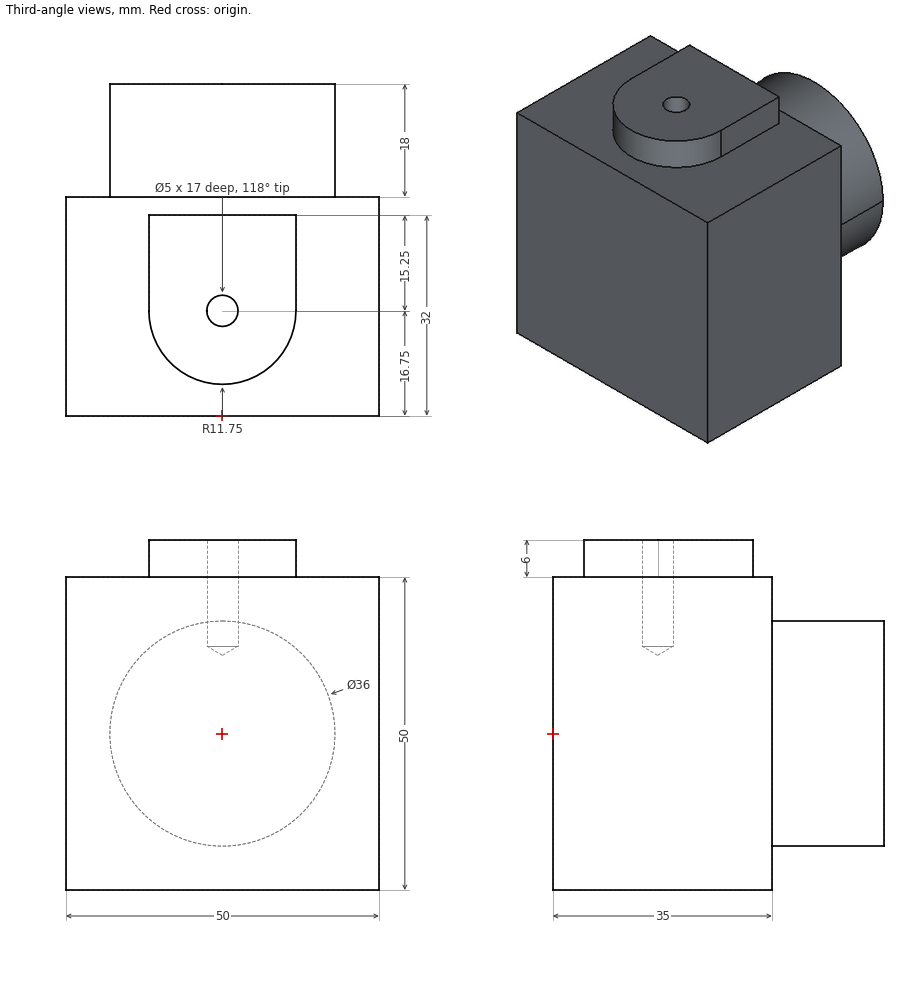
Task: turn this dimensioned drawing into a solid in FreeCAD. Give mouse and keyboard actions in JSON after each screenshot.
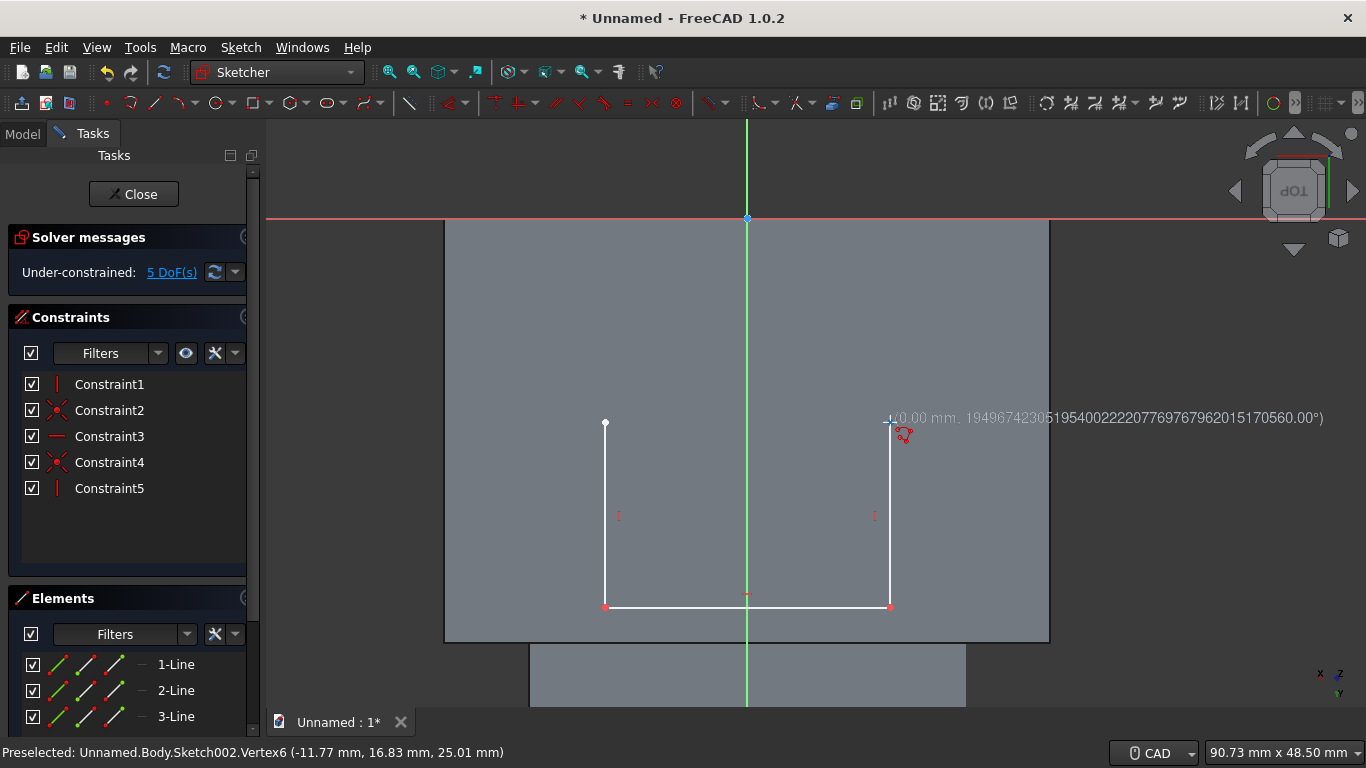
{"action": "key", "text": "g 3 a"}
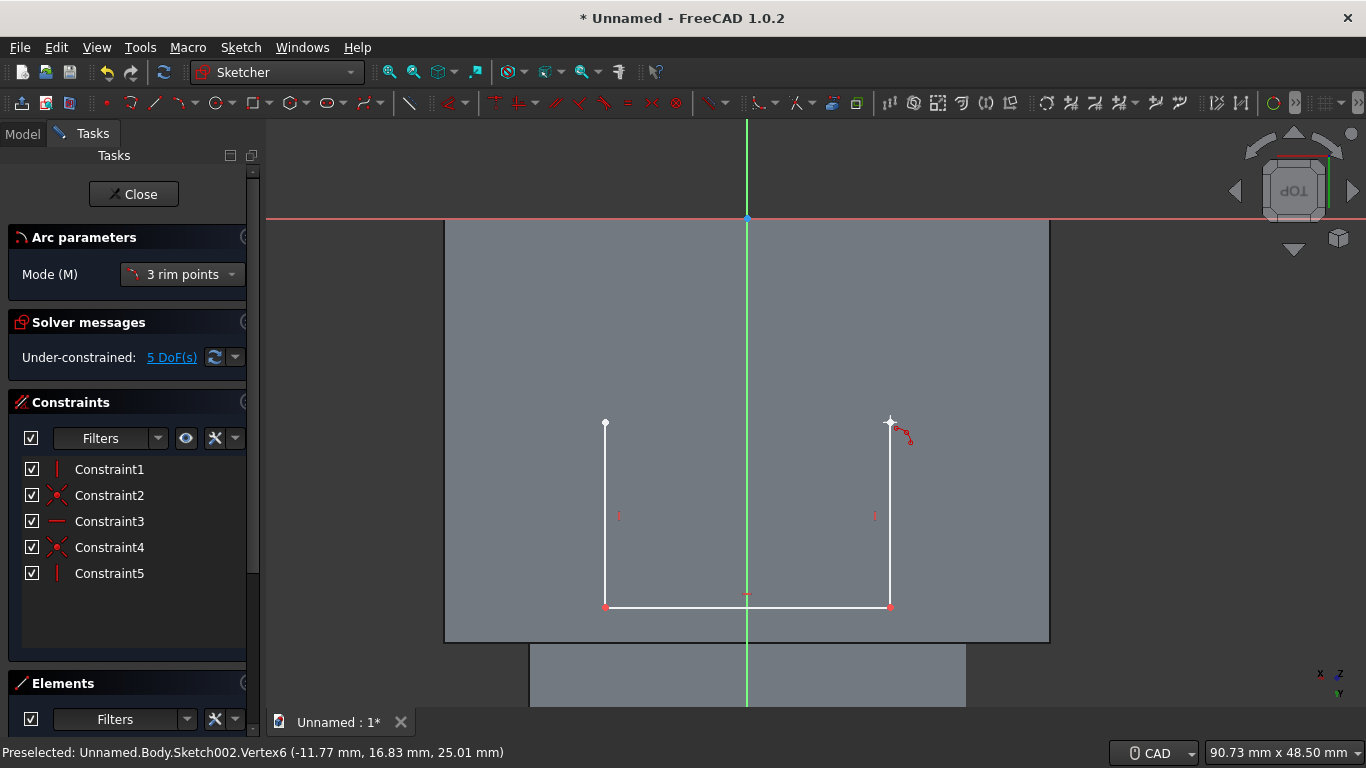
{"action": "left_click", "coordinate": [890, 423]}
{"action": "left_click", "coordinate": [605, 423]}
{"action": "left_click", "coordinate": [791, 287]}
{"action": "key", "text": "Escape"}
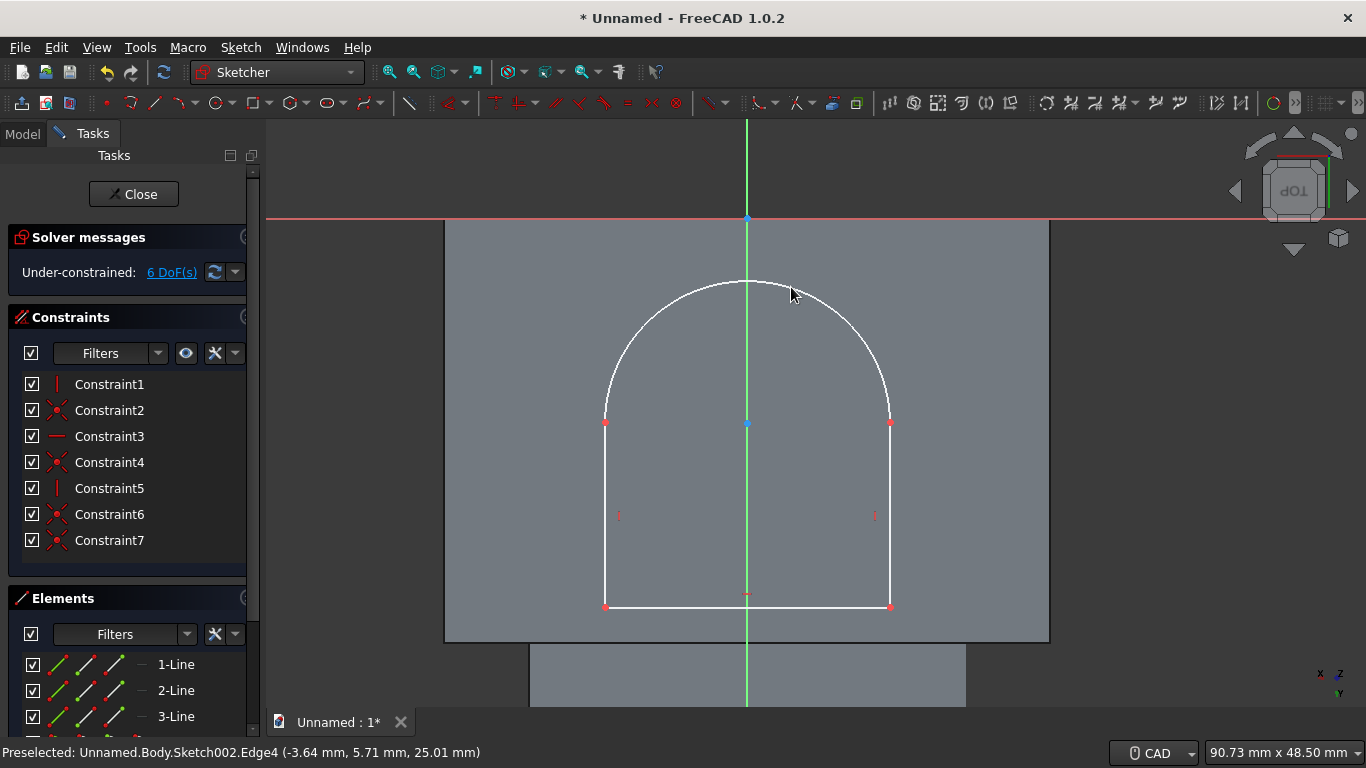
{"action": "left_click", "coordinate": [605, 479]}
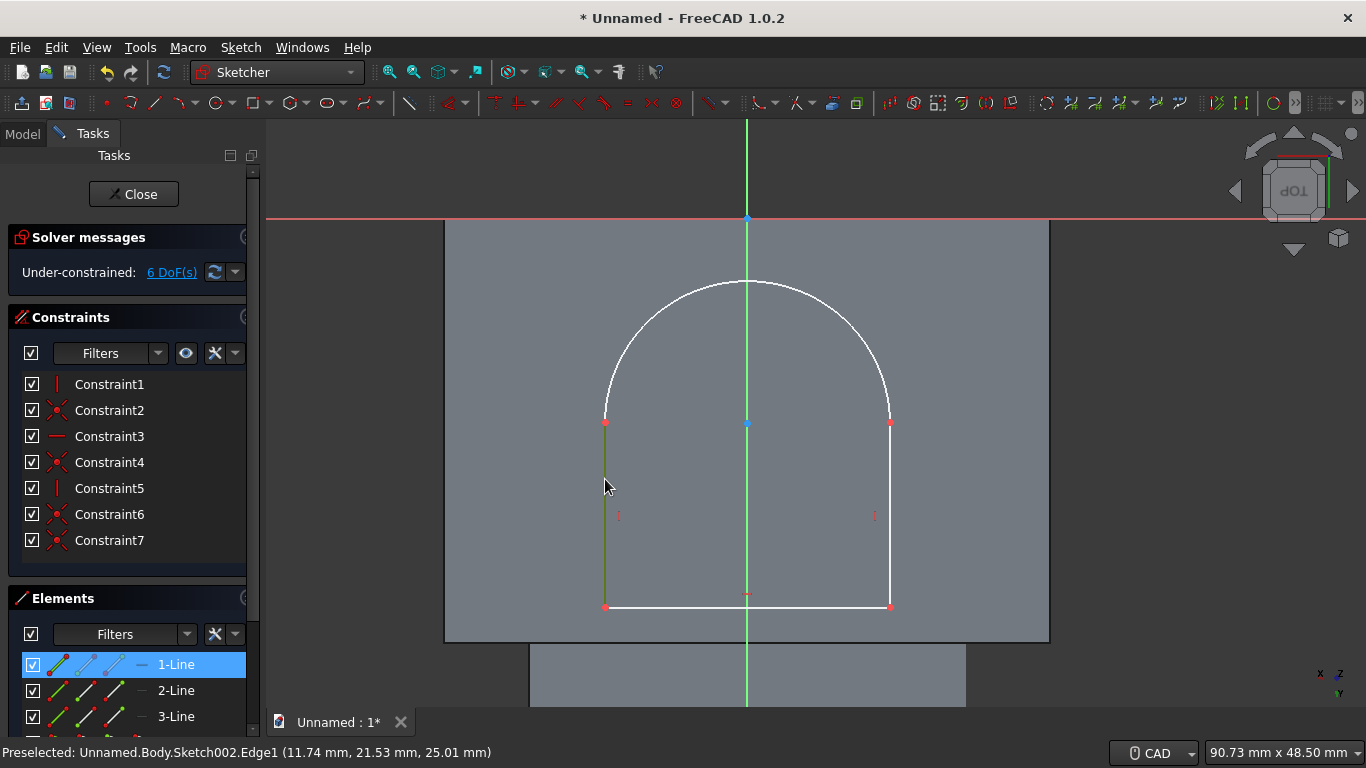
{"action": "left_click", "coordinate": [831, 308]}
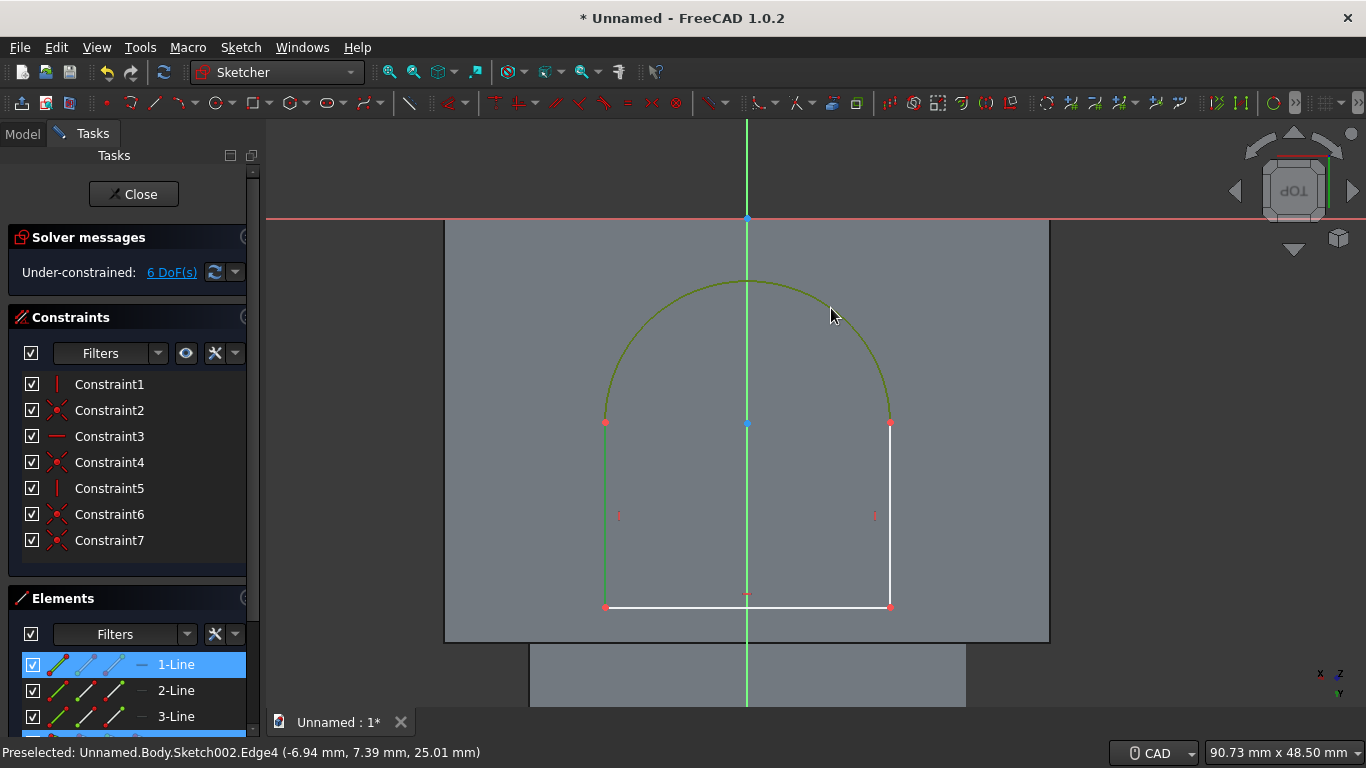
{"action": "key", "text": "t"}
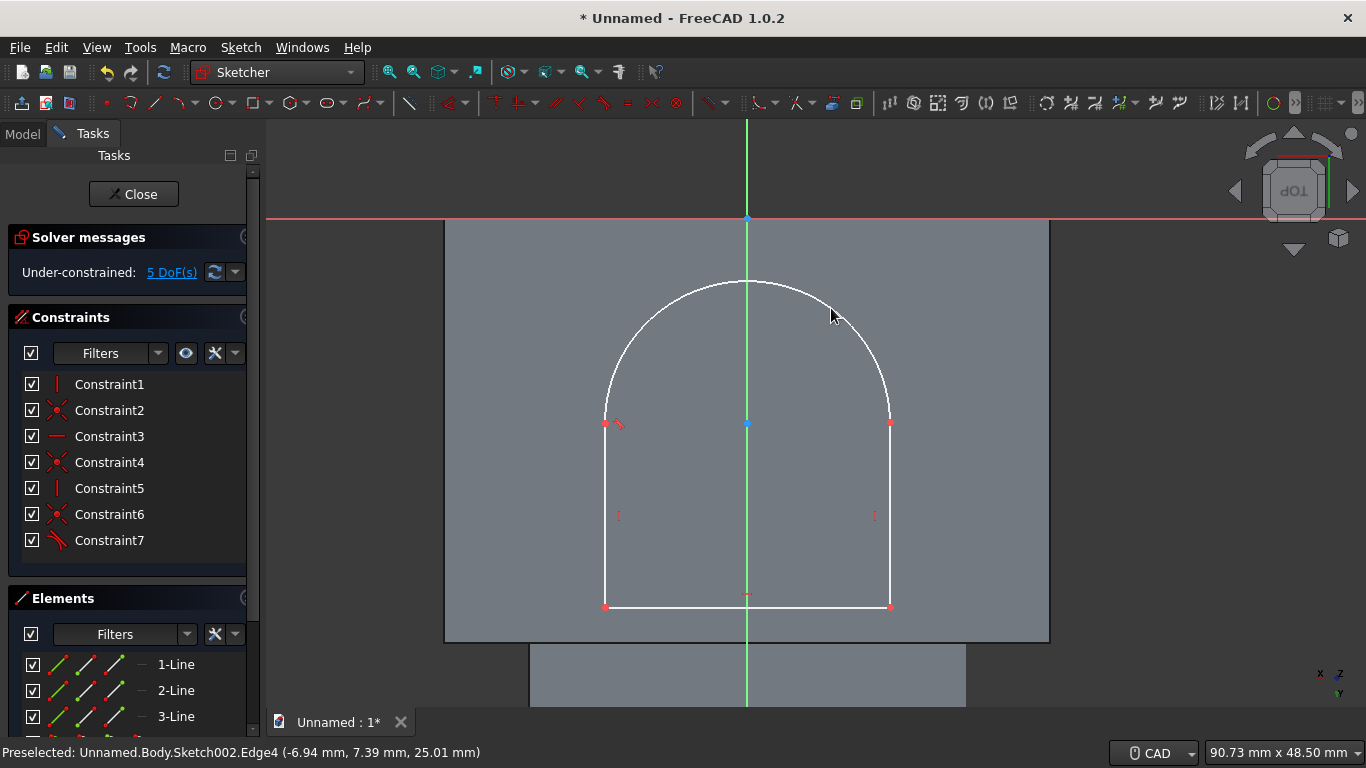
{"action": "left_click", "coordinate": [890, 553]}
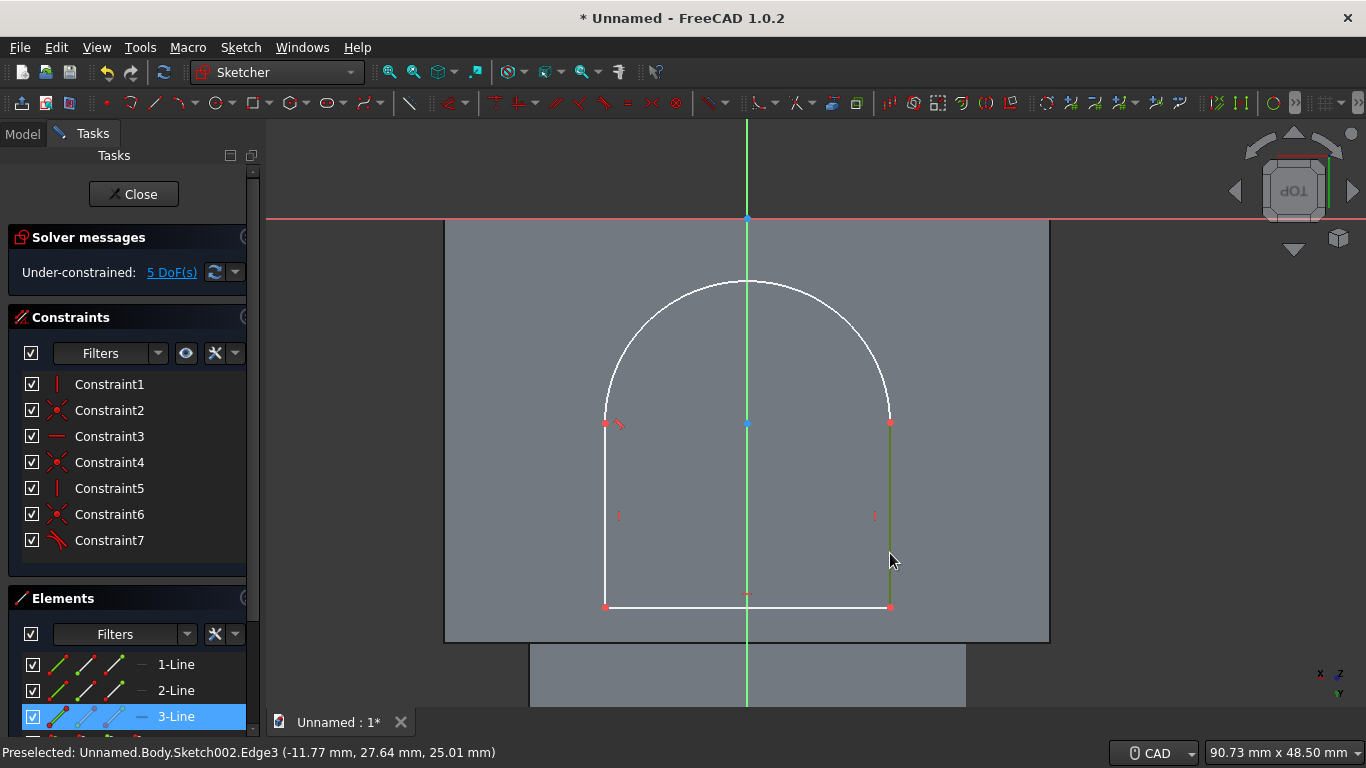
{"action": "left_click", "coordinate": [831, 308]}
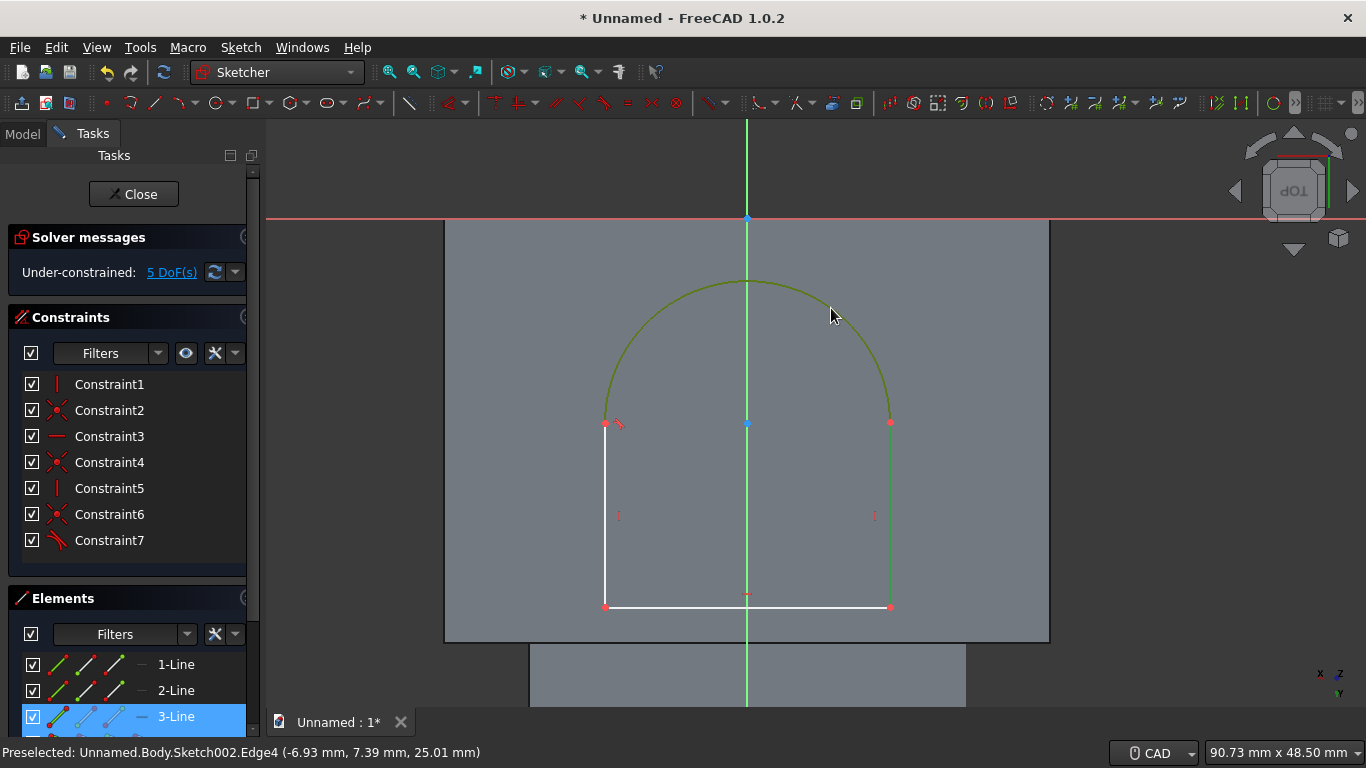
{"action": "key", "text": "t"}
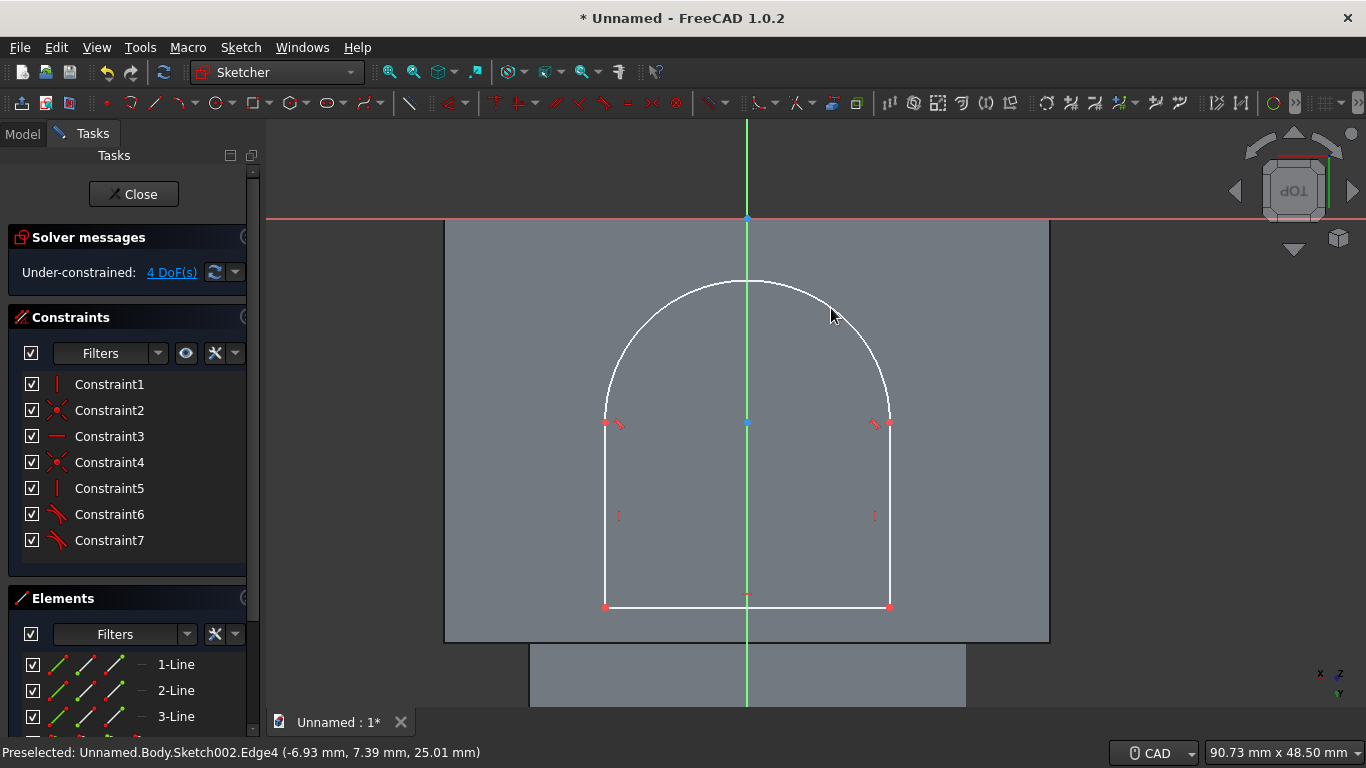
{"action": "left_click", "coordinate": [747, 423]}